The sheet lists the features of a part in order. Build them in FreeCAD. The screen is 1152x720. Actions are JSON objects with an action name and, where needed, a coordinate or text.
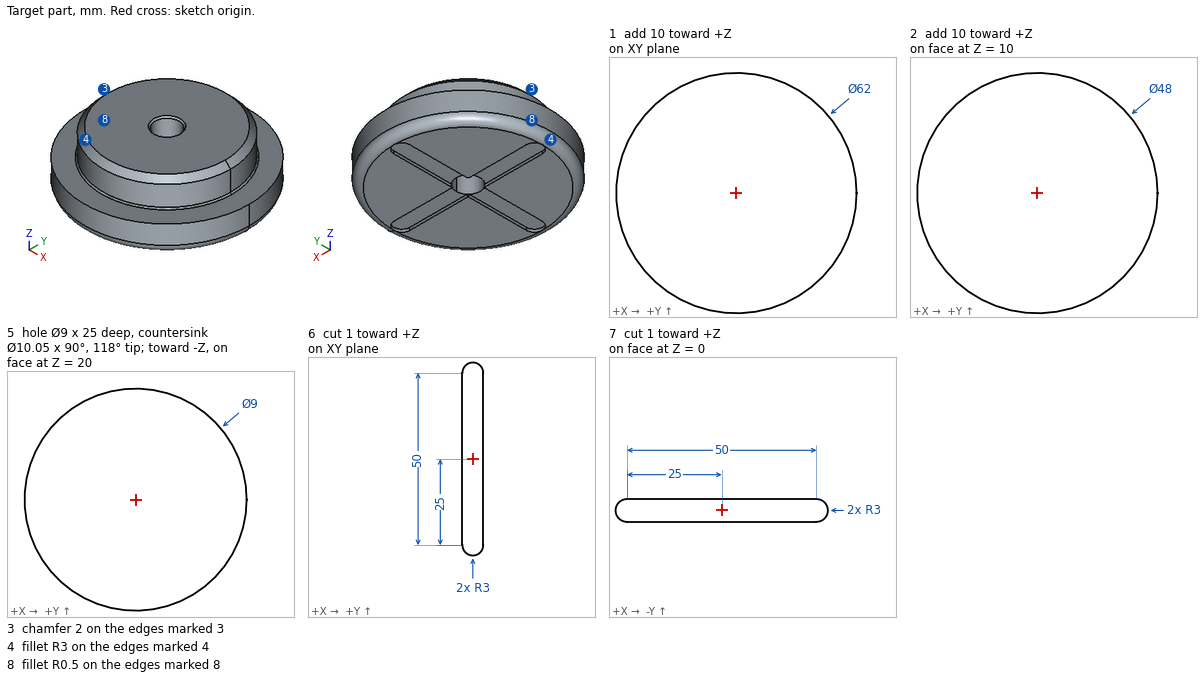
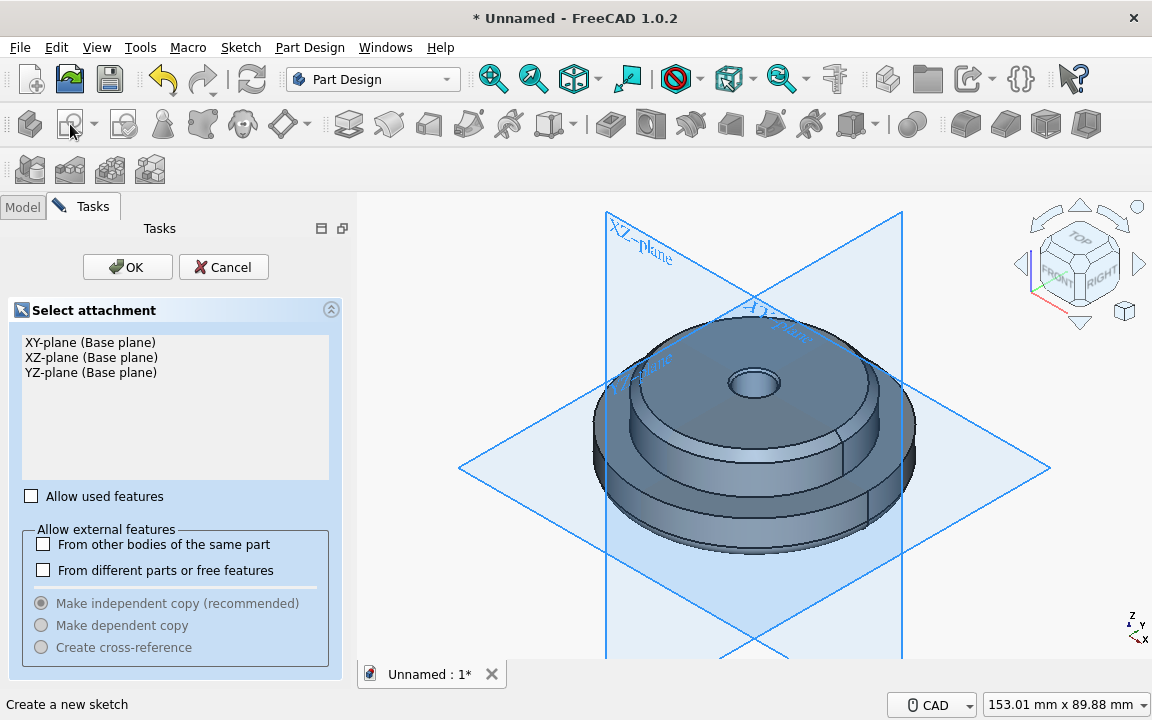
{"action": "left_click", "coordinate": [82, 342]}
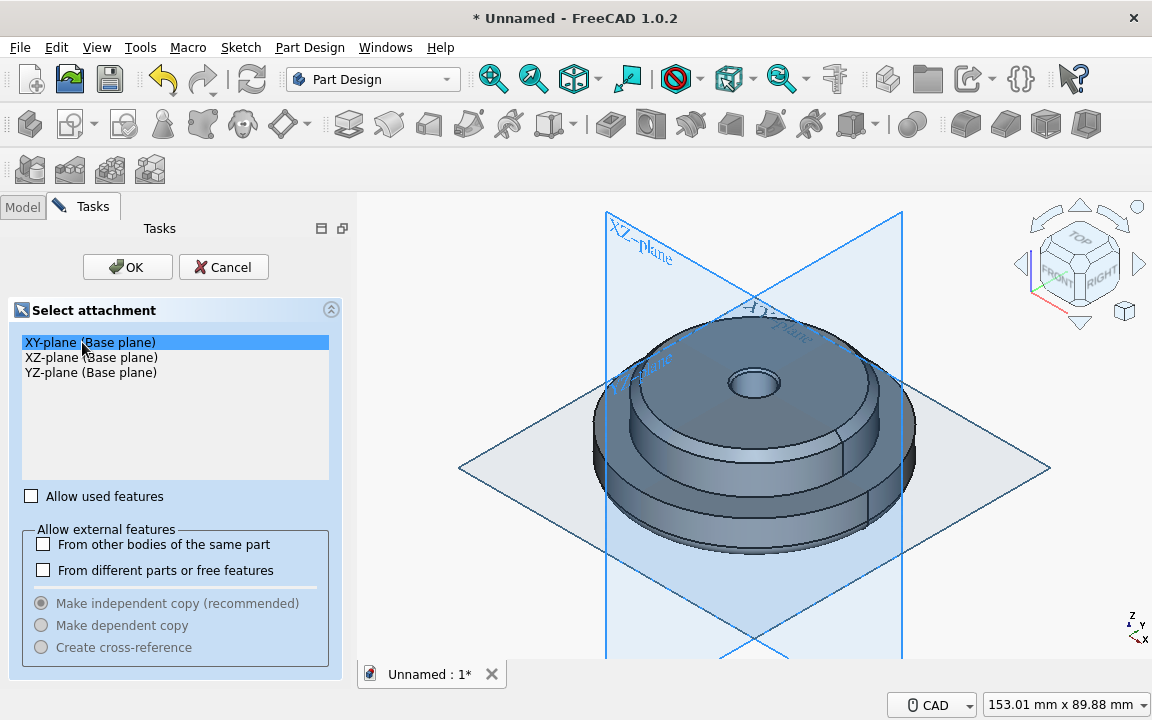
{"action": "left_click", "coordinate": [128, 267]}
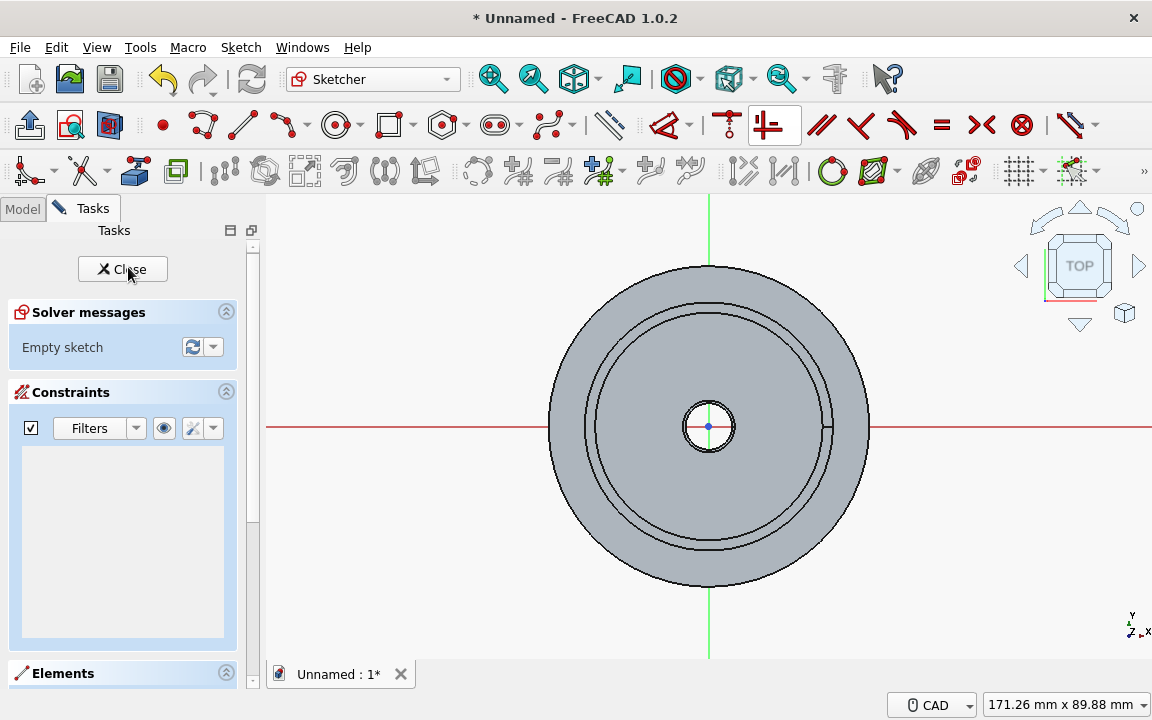
{"action": "left_click", "coordinate": [110, 126]}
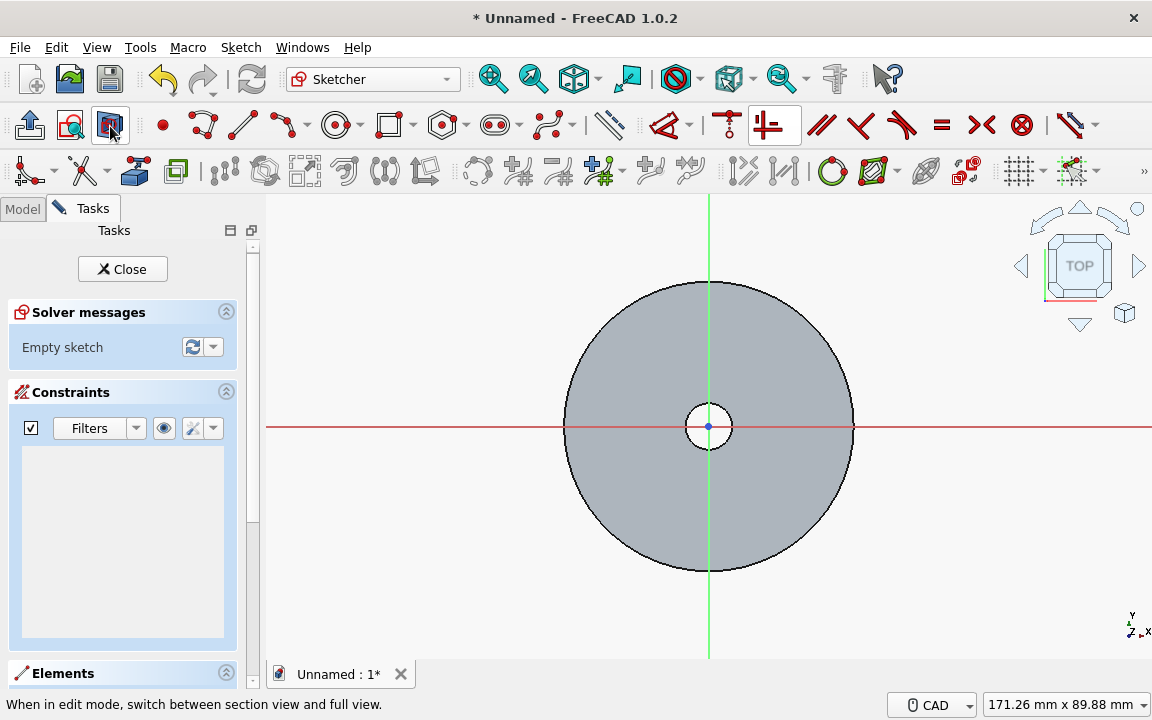
{"action": "key", "text": "g s"}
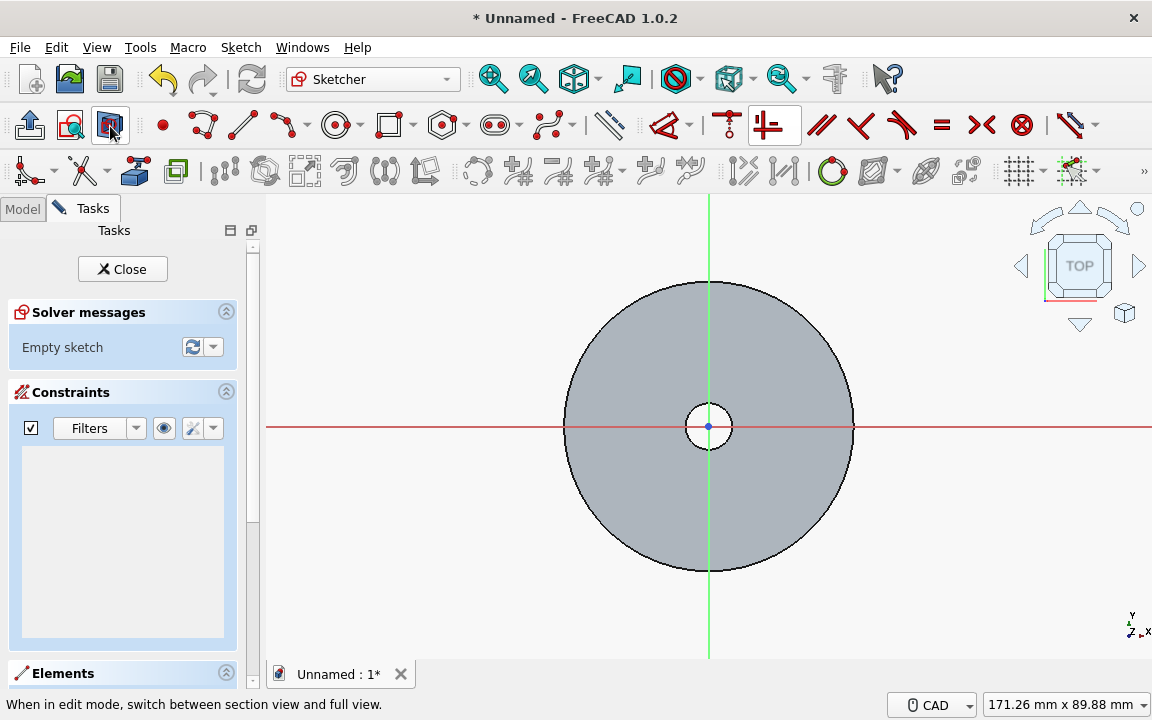
{"action": "scroll", "coordinate": [709, 556], "scroll_direction": "up", "scroll_amount": 2}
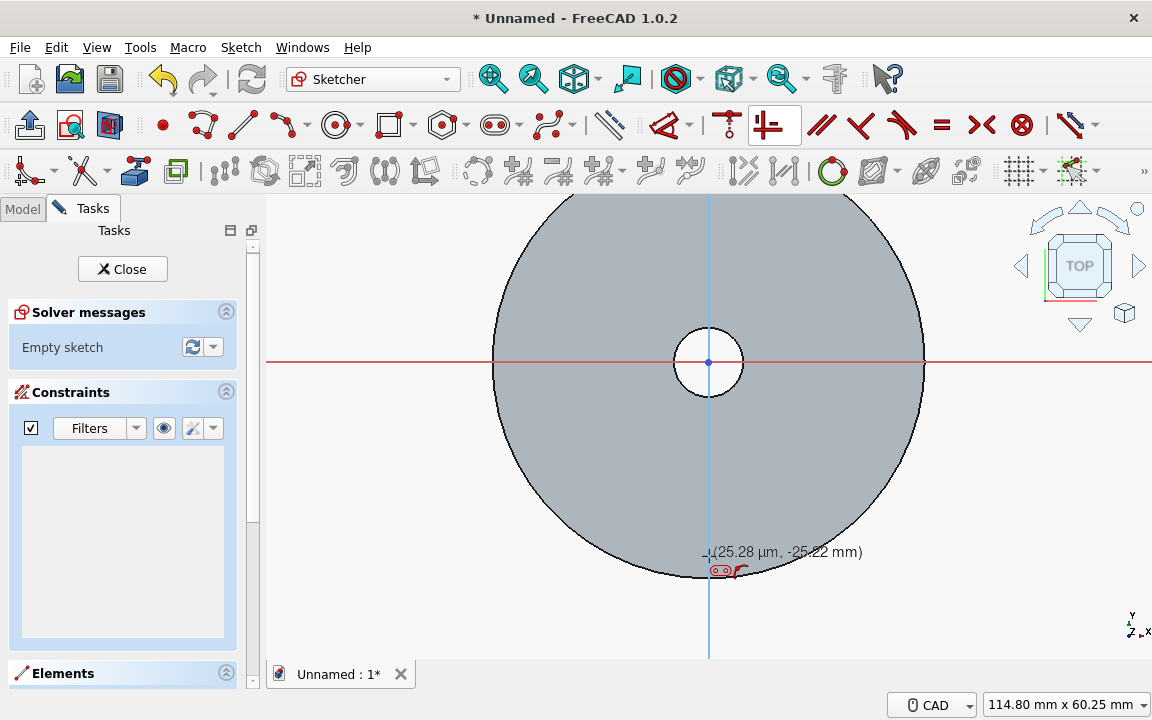
{"action": "left_click", "coordinate": [709, 555]}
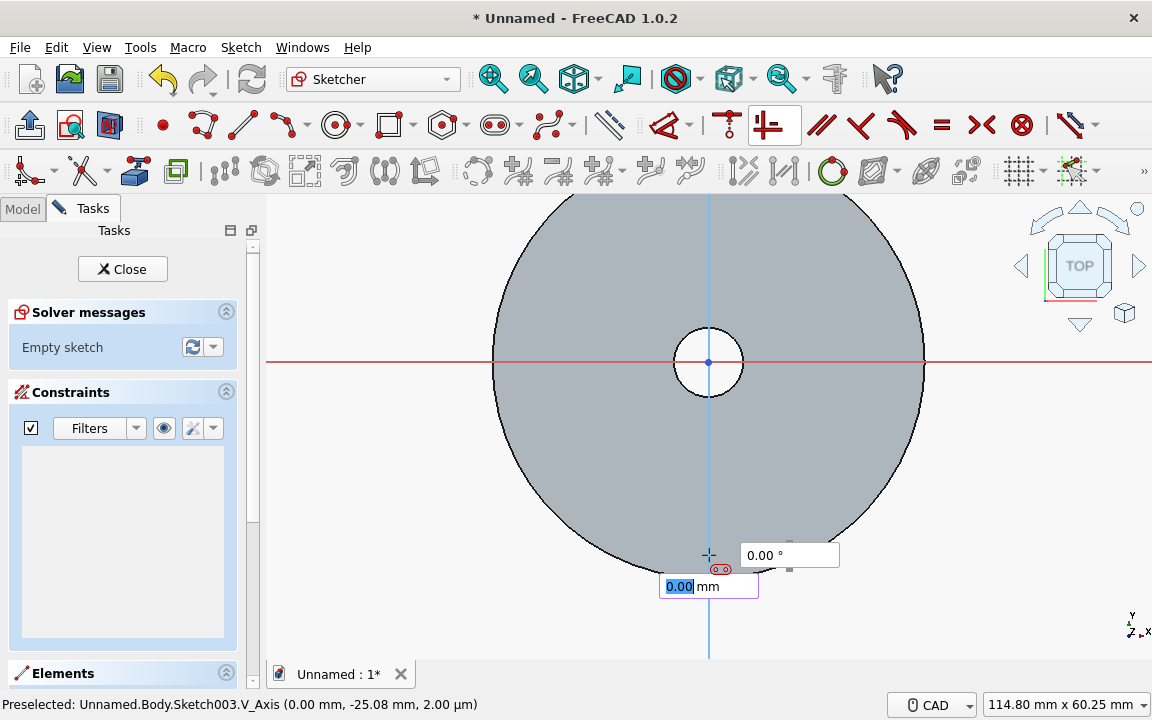
{"action": "scroll", "coordinate": [502, 557], "scroll_direction": "down", "scroll_amount": 2}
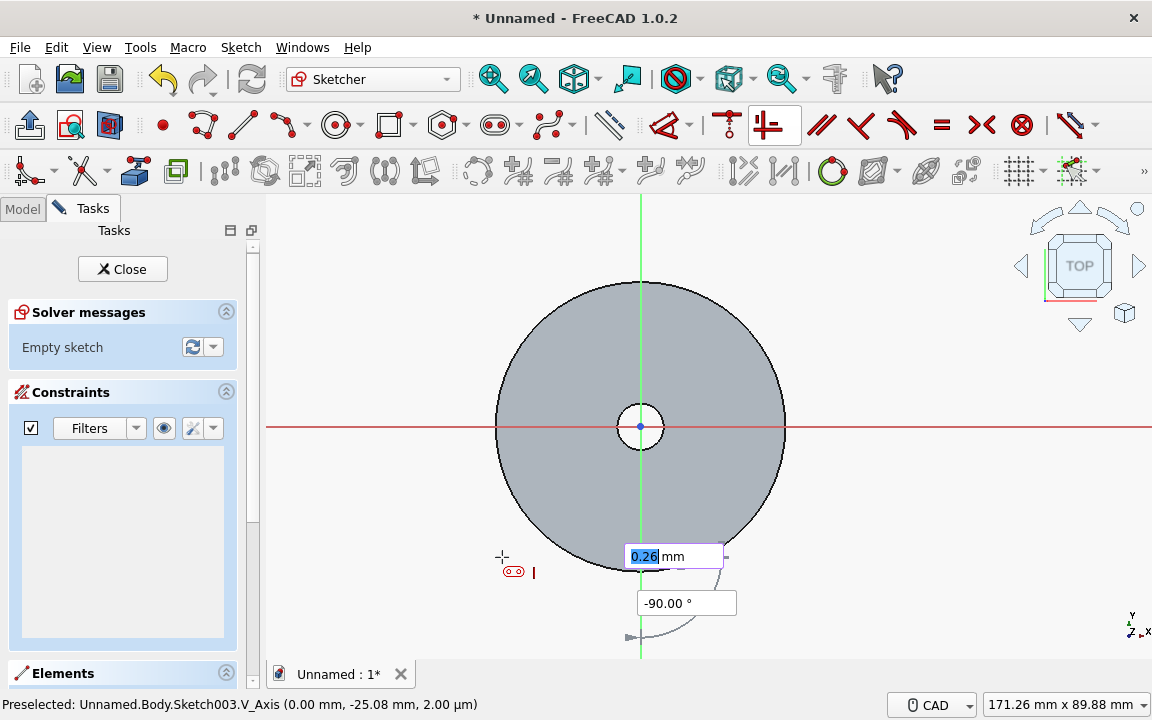
{"action": "left_click", "coordinate": [650, 297]}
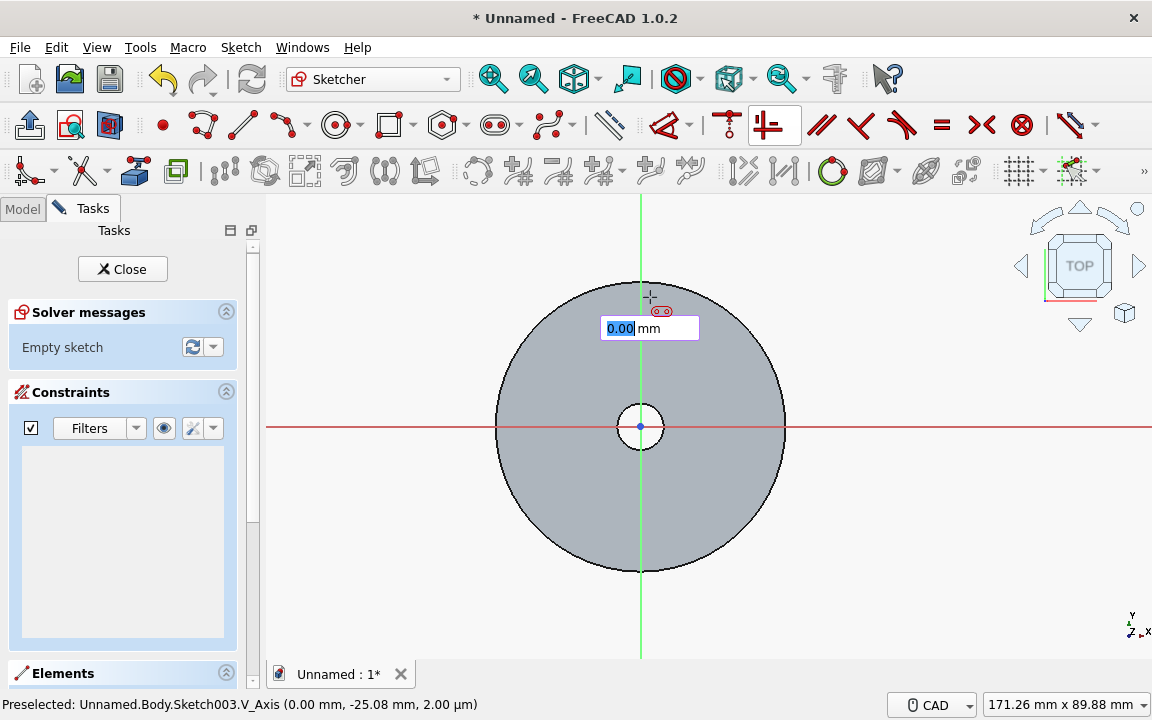
{"action": "left_click", "coordinate": [656, 388]}
{"action": "key", "text": "Escape"}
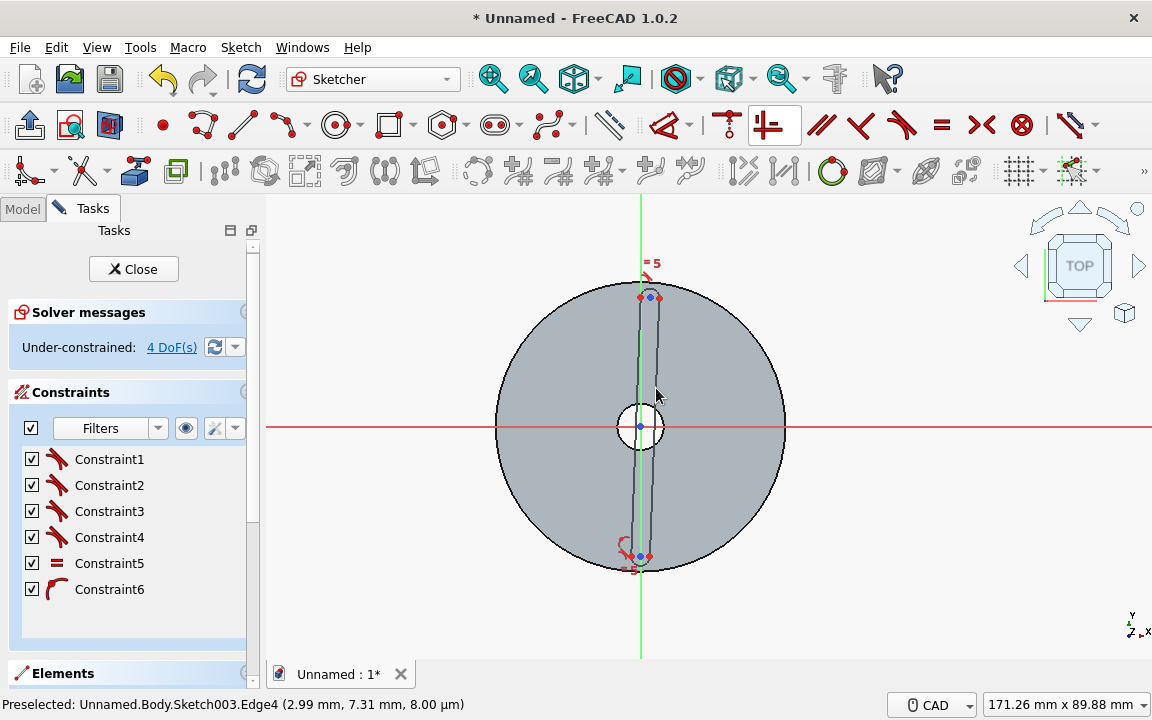
{"action": "left_click", "coordinate": [638, 375]}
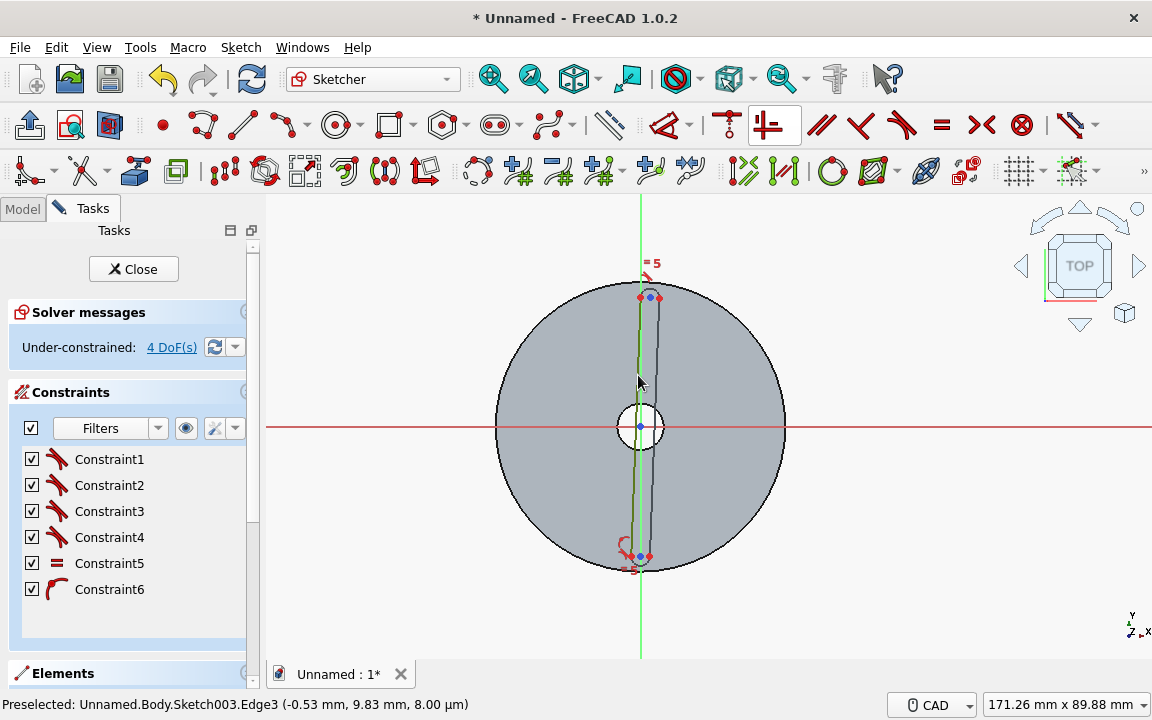
{"action": "left_click", "coordinate": [796, 126]}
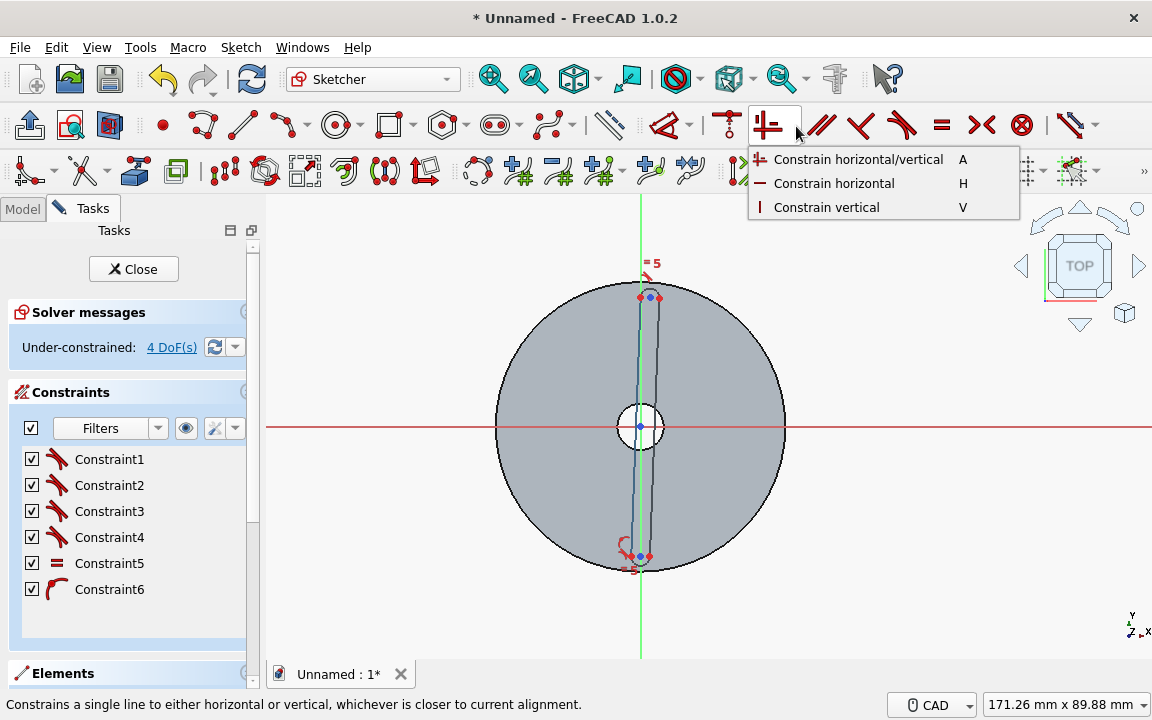
{"action": "left_click", "coordinate": [884, 207]}